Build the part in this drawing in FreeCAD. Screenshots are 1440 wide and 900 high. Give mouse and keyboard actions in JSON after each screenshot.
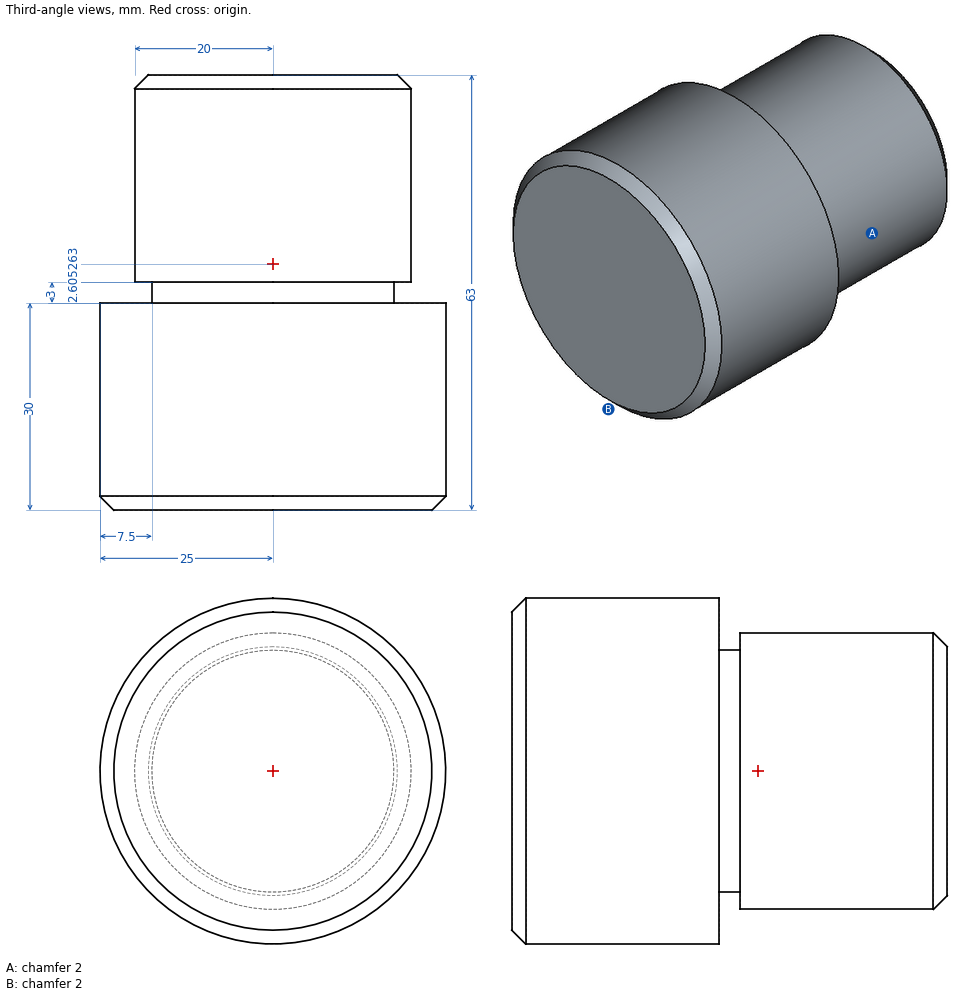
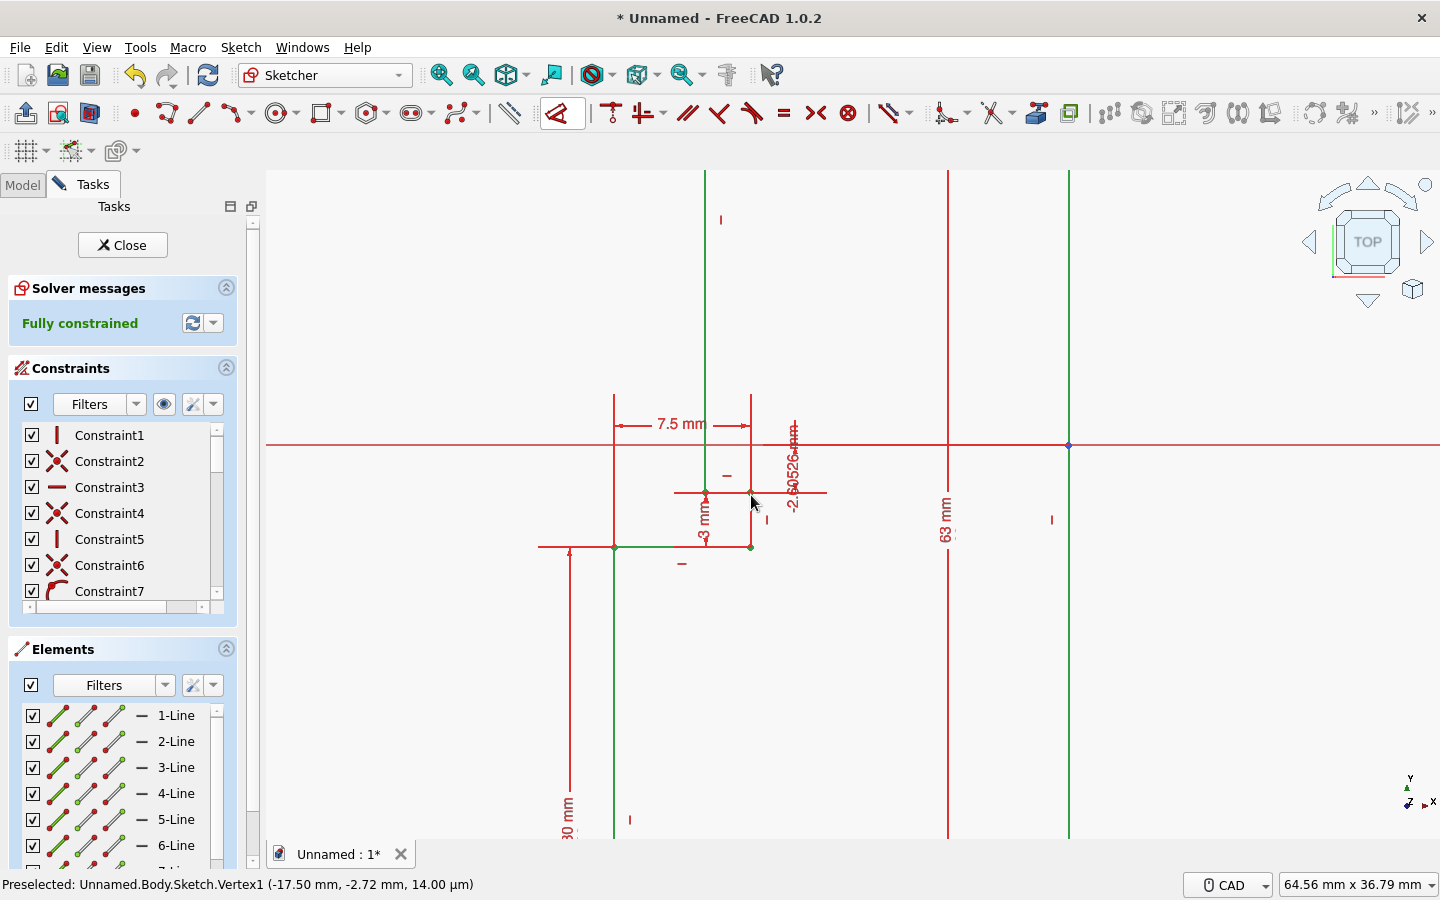
{"action": "left_click", "coordinate": [123, 245]}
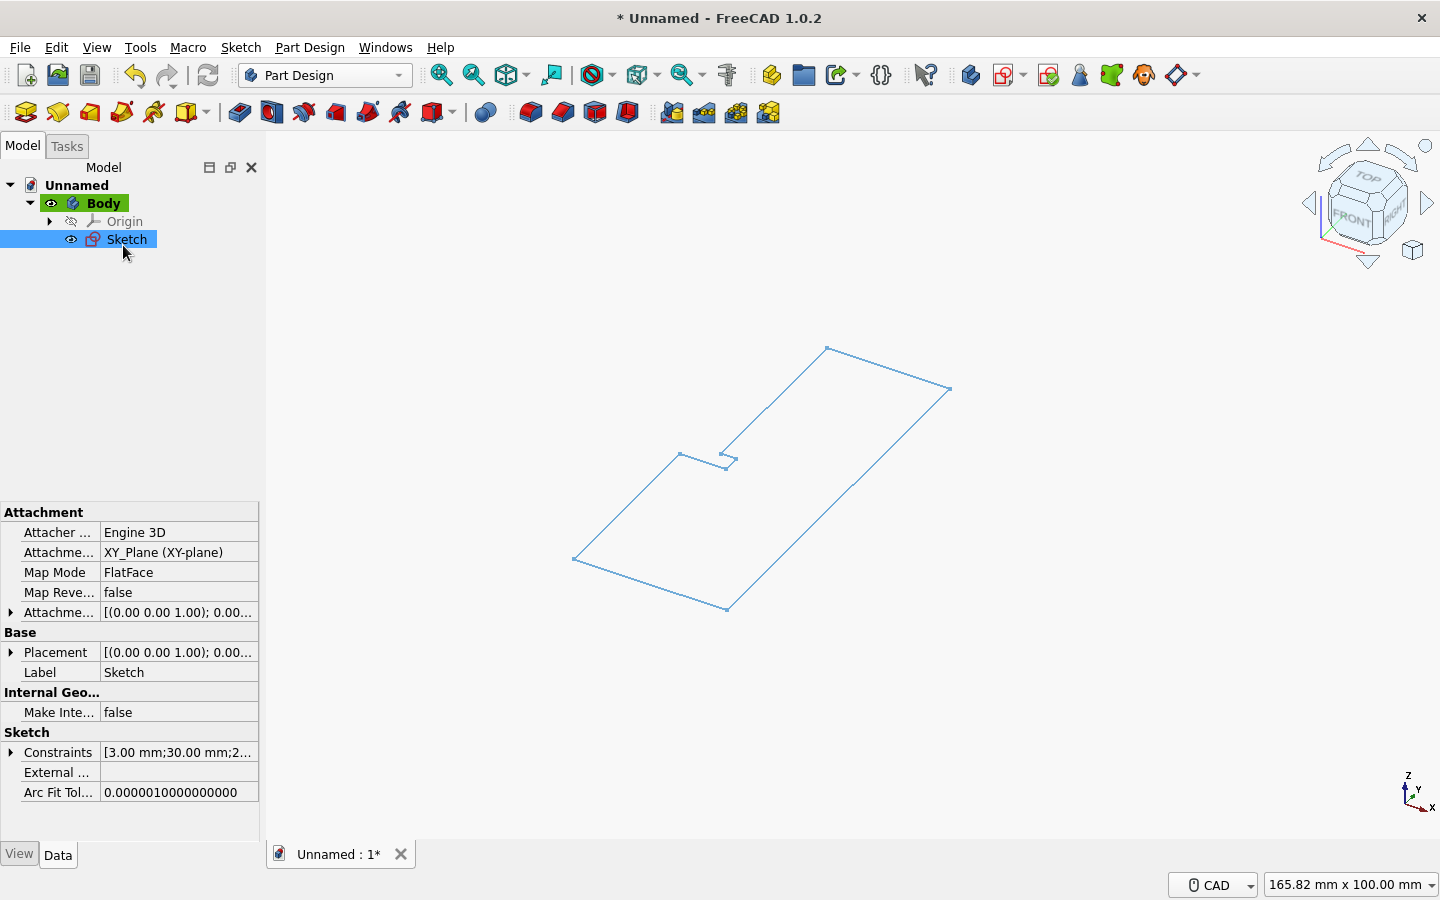
{"action": "left_click", "coordinate": [58, 112]}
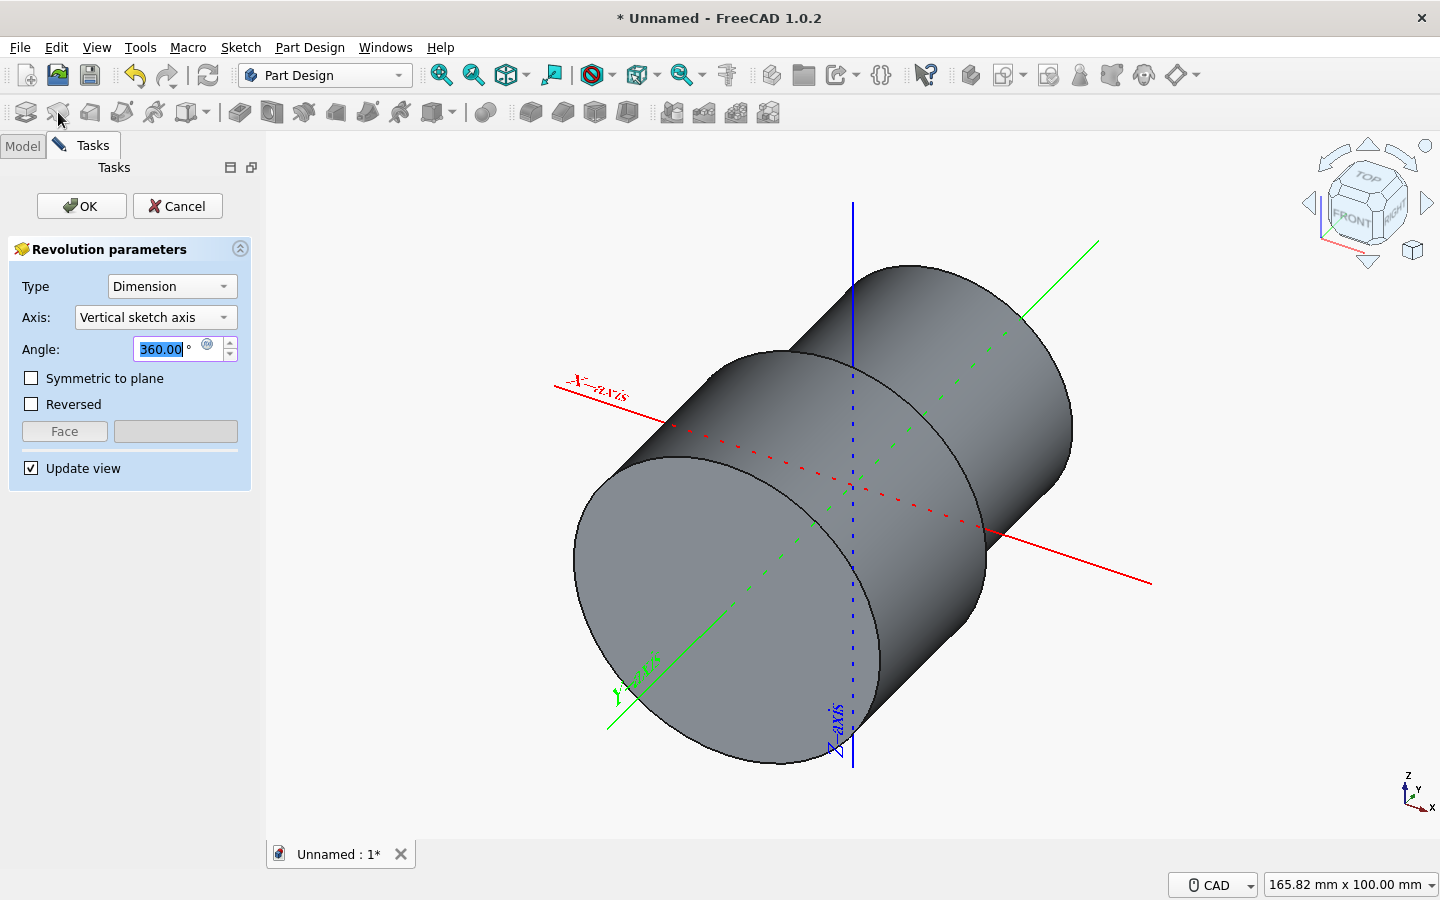
{"action": "left_click", "coordinate": [82, 206]}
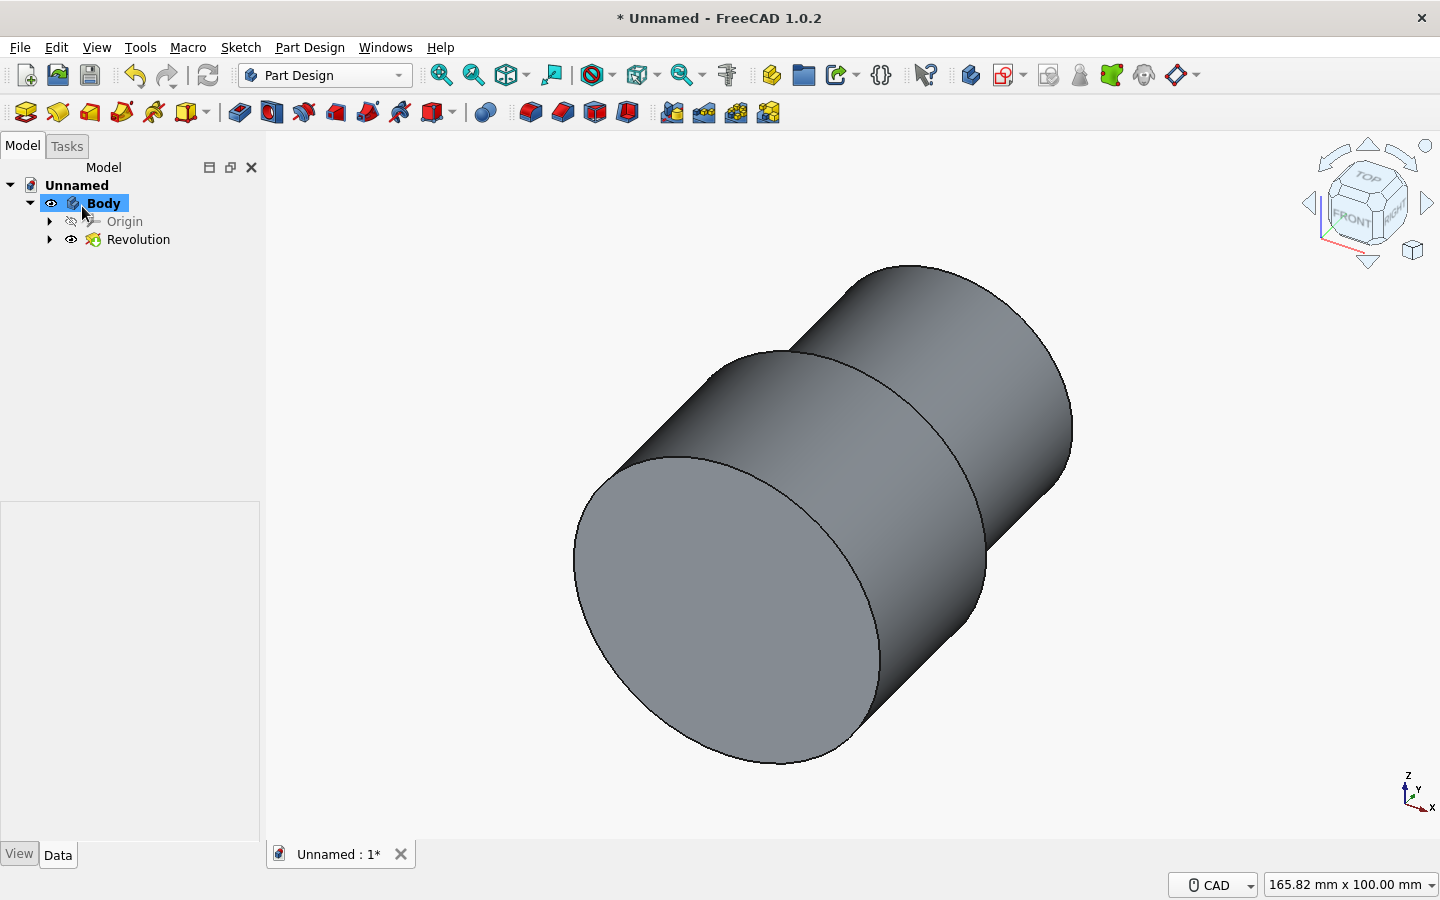
{"action": "key", "text": "0"}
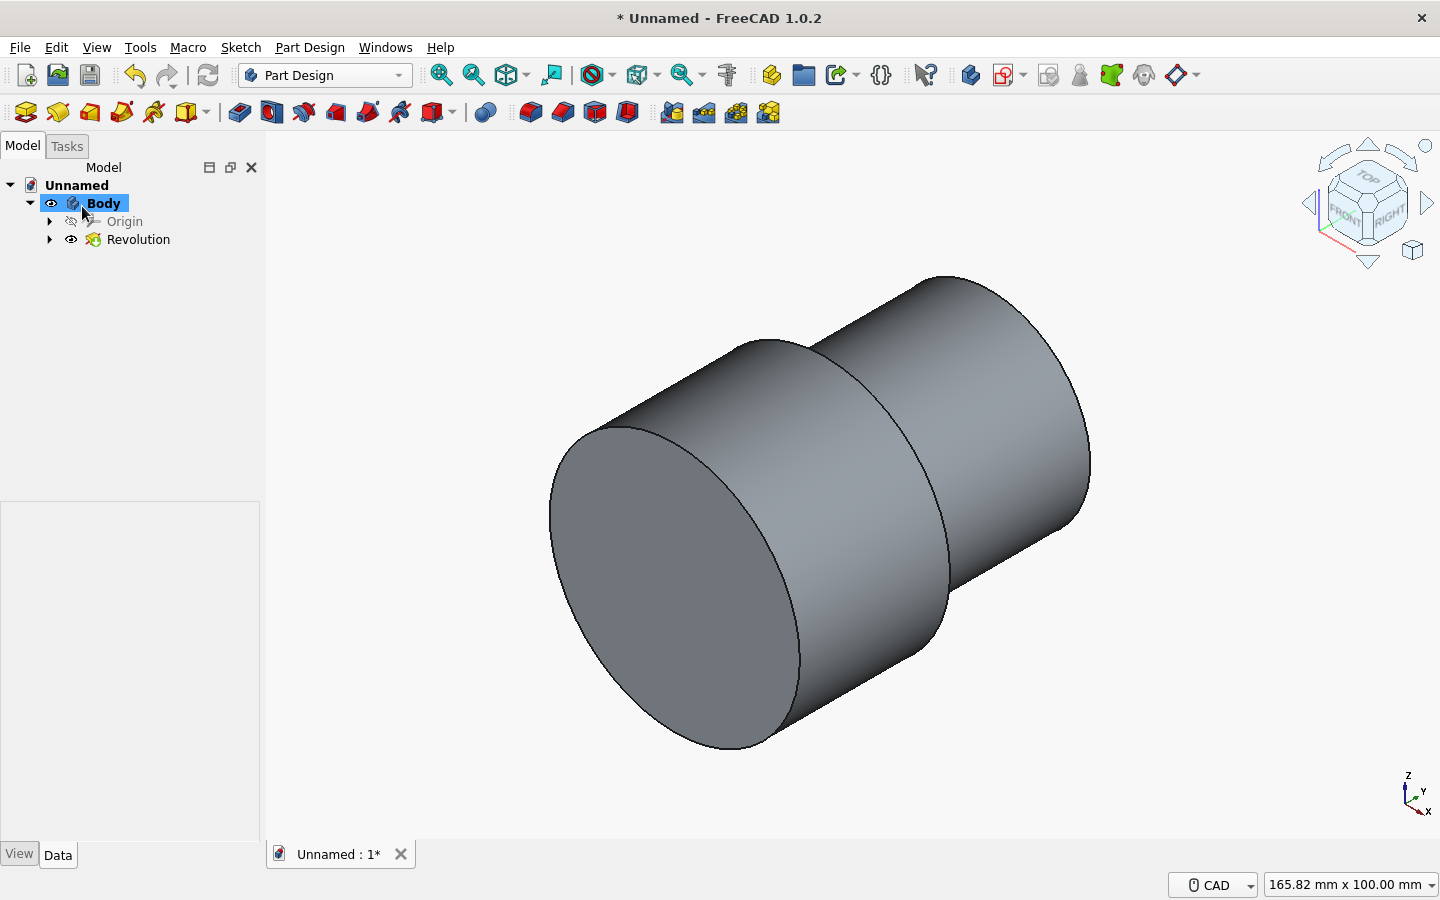
{"action": "key", "text": "2"}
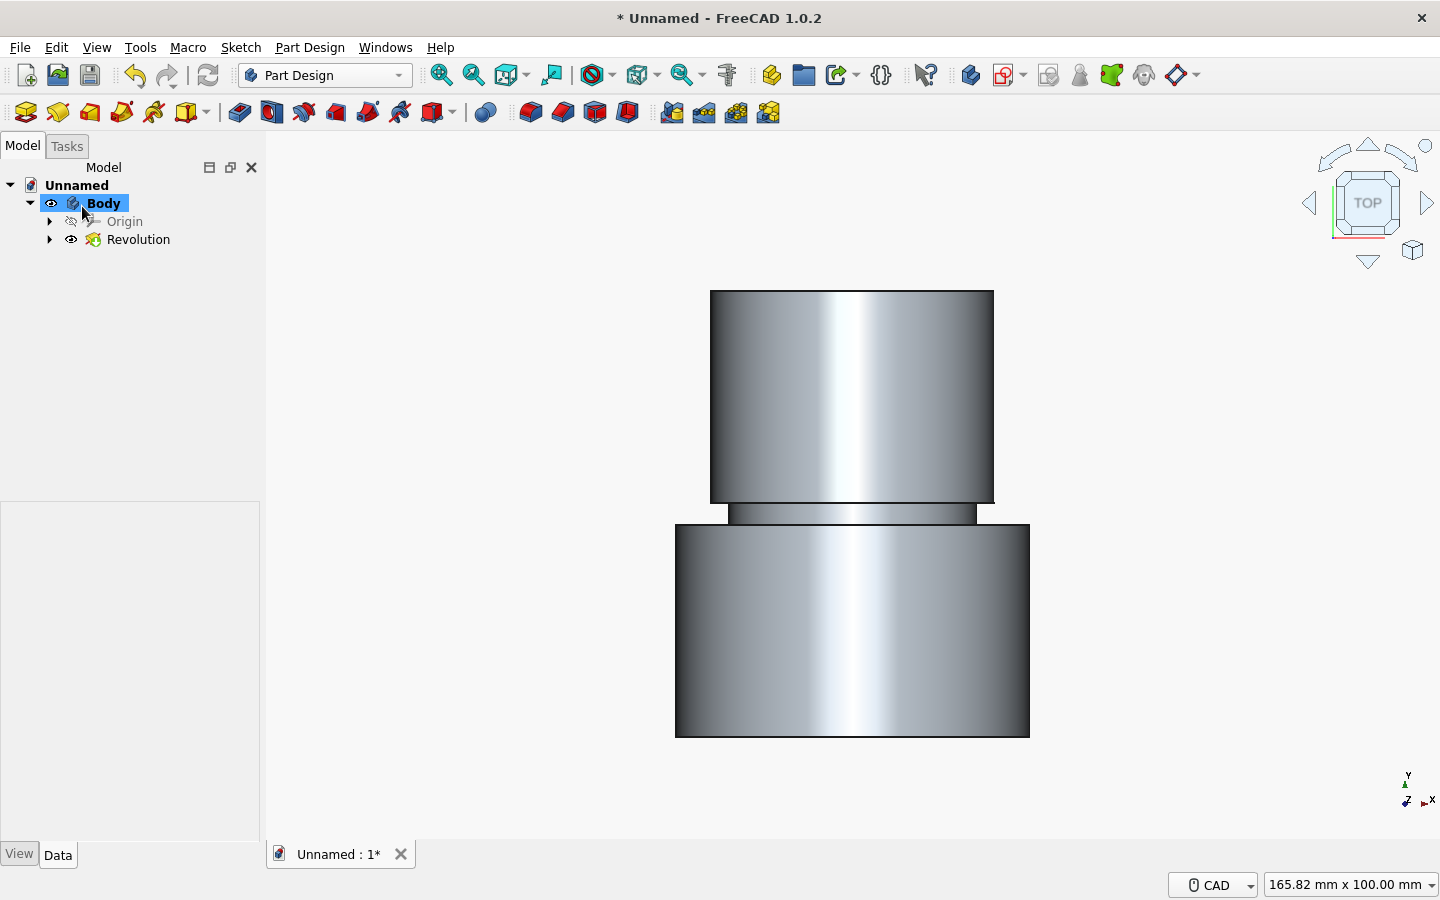
{"action": "left_click", "coordinate": [968, 290]}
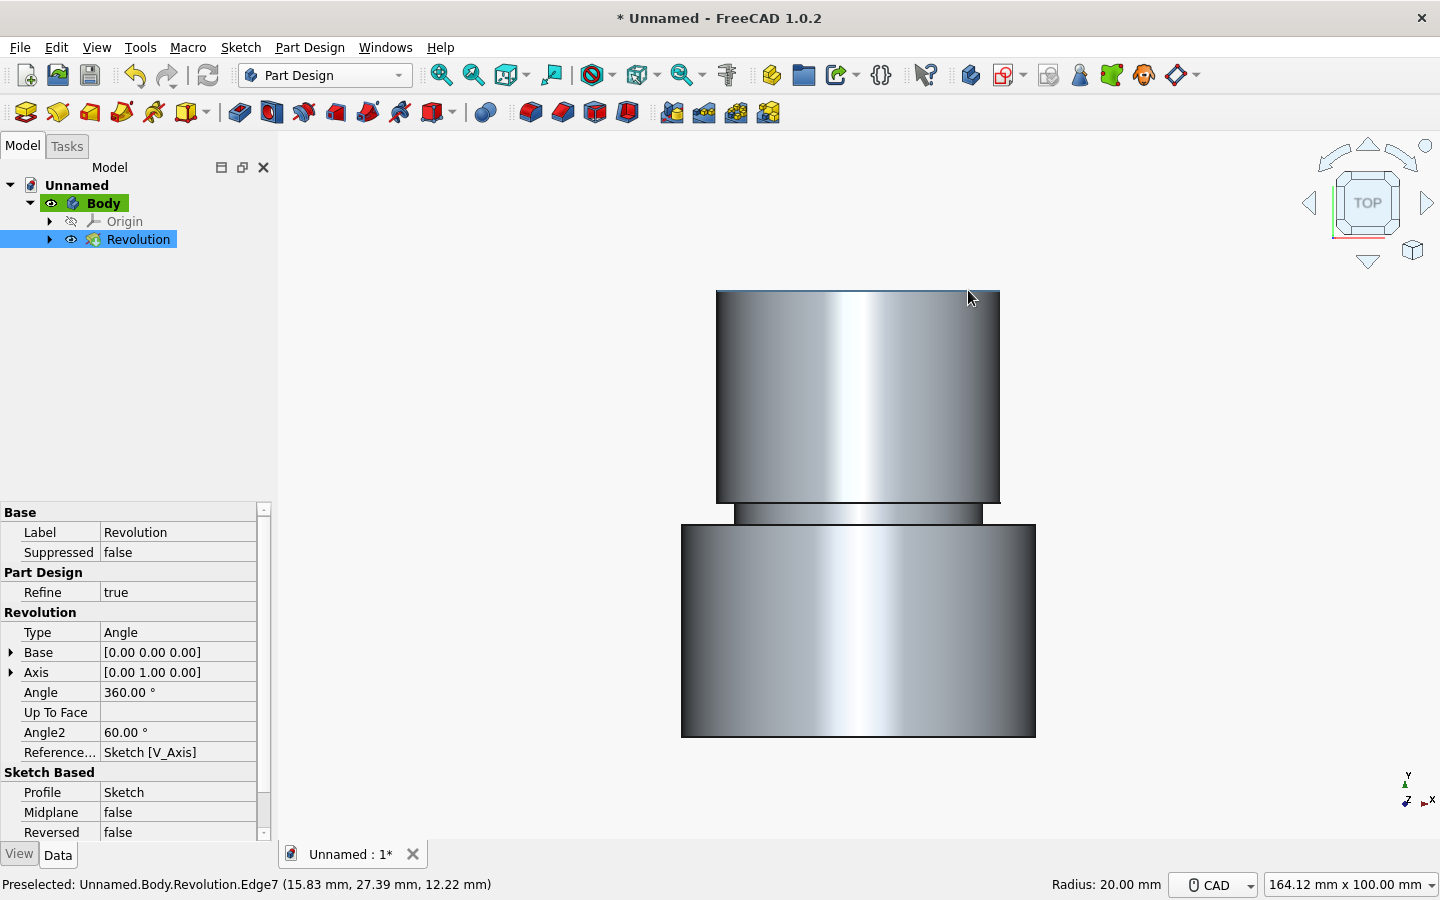
{"action": "left_click", "coordinate": [564, 112]}